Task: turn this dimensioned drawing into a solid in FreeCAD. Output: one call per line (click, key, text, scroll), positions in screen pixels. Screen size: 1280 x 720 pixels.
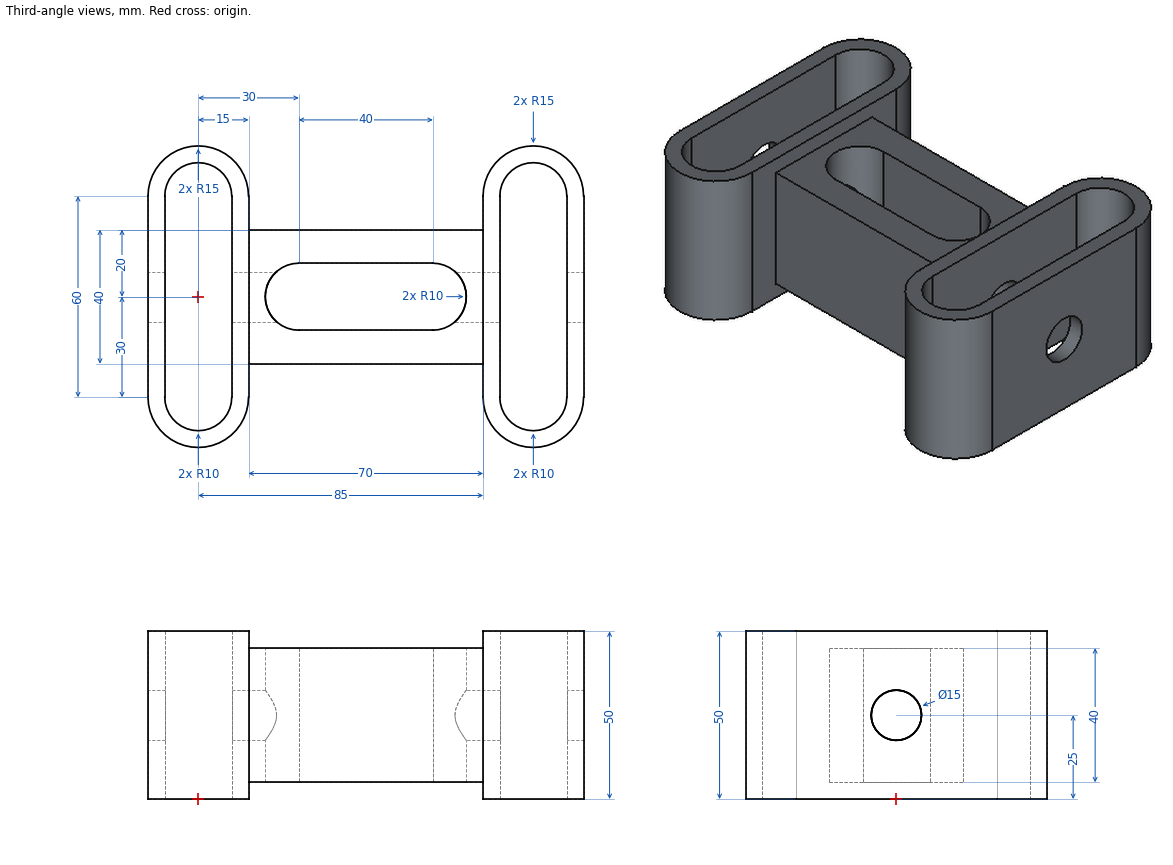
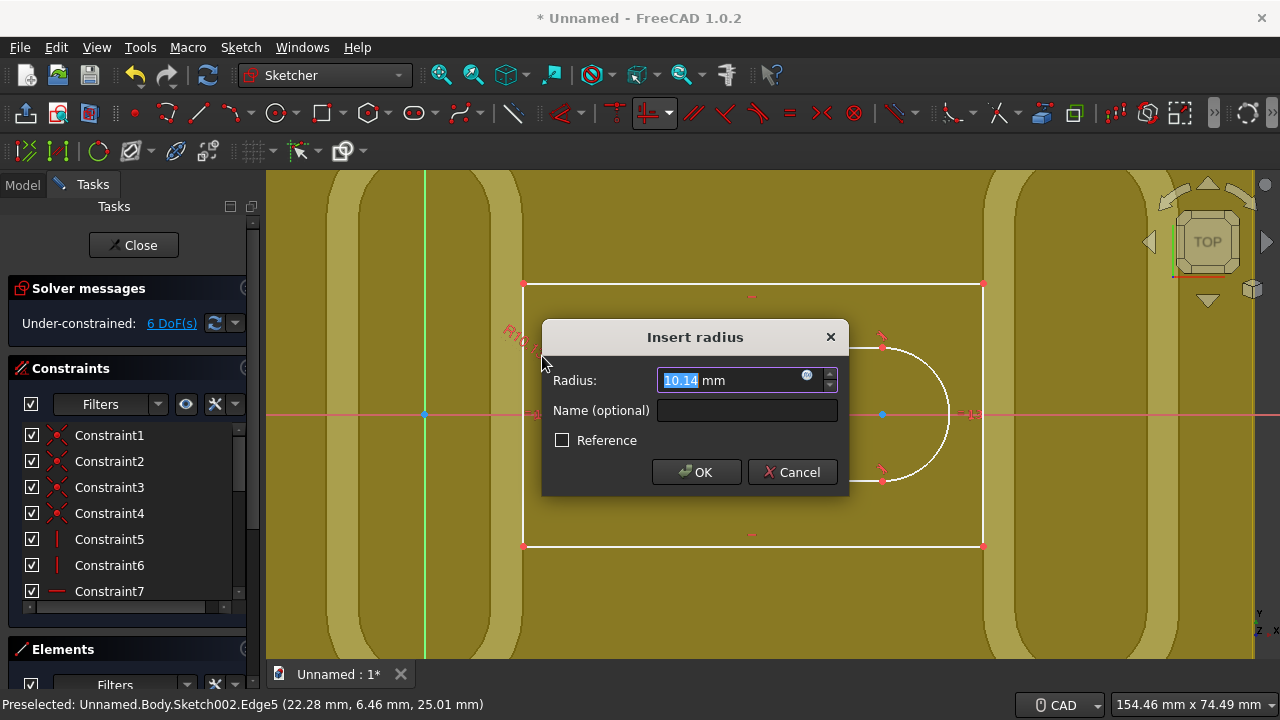
text(10)
key(Return)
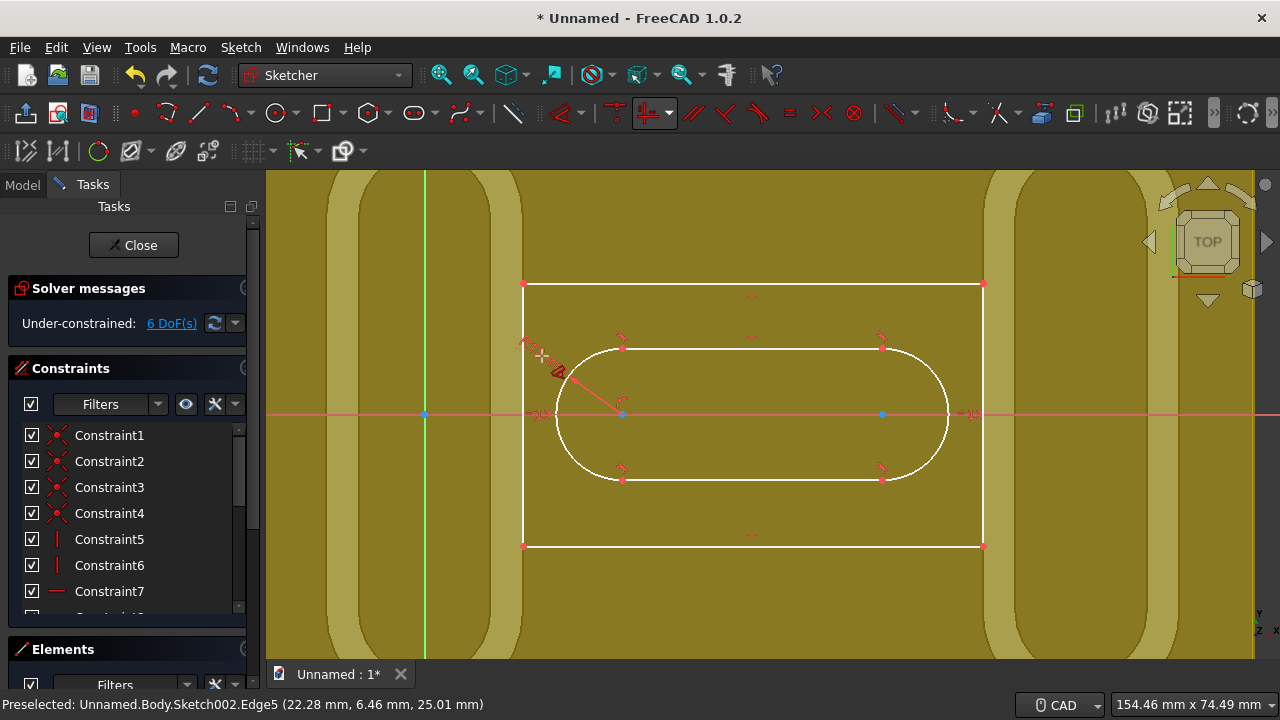
click(523, 363)
click(489, 476)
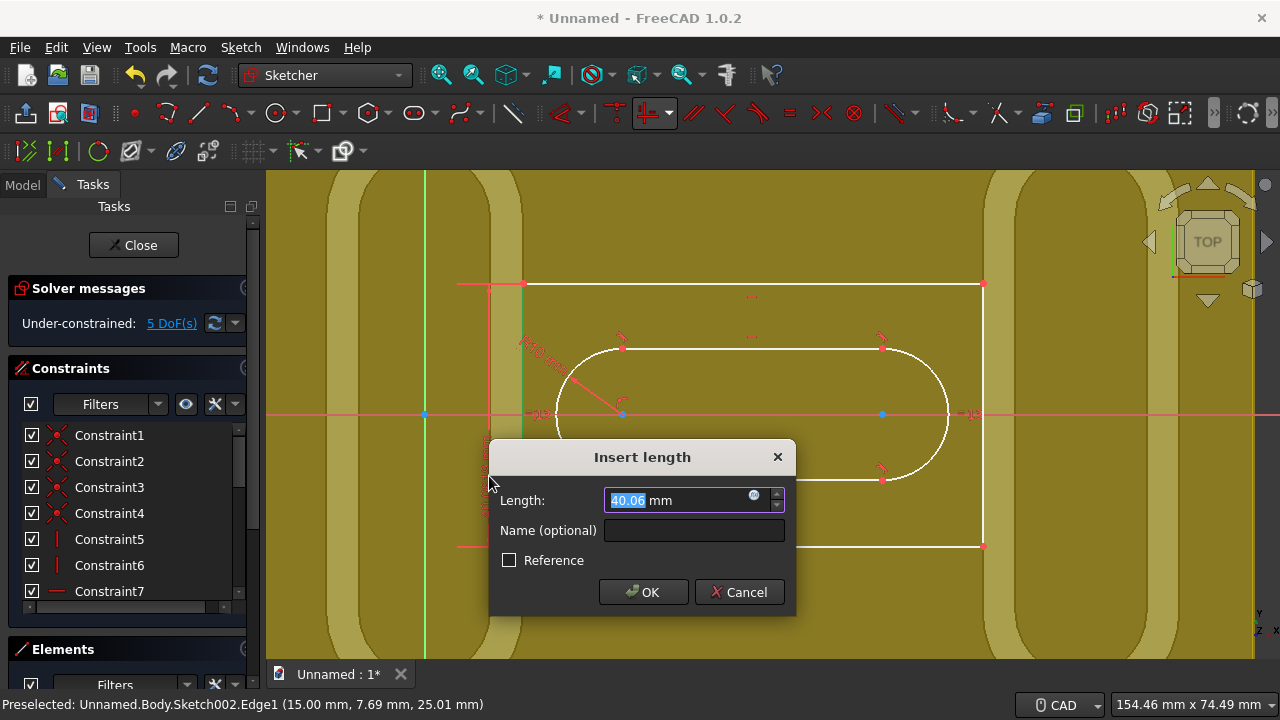
text(40)
key(Return)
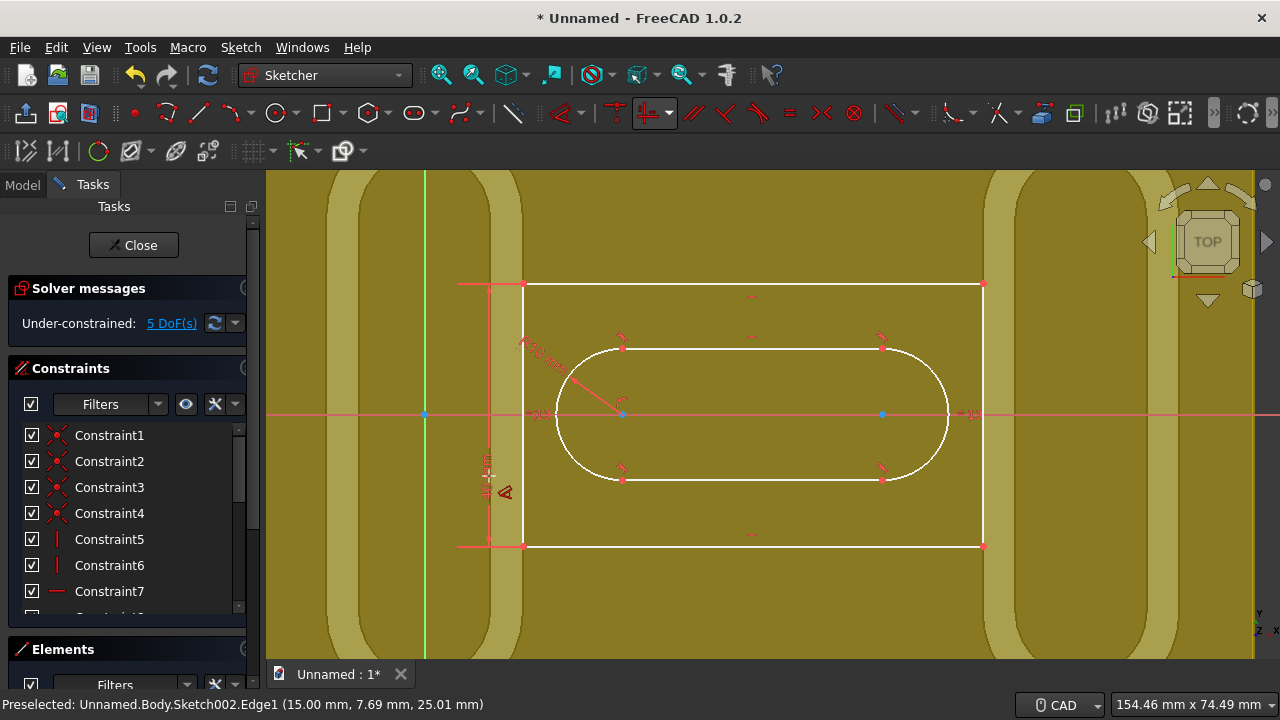
click(661, 547)
click(753, 581)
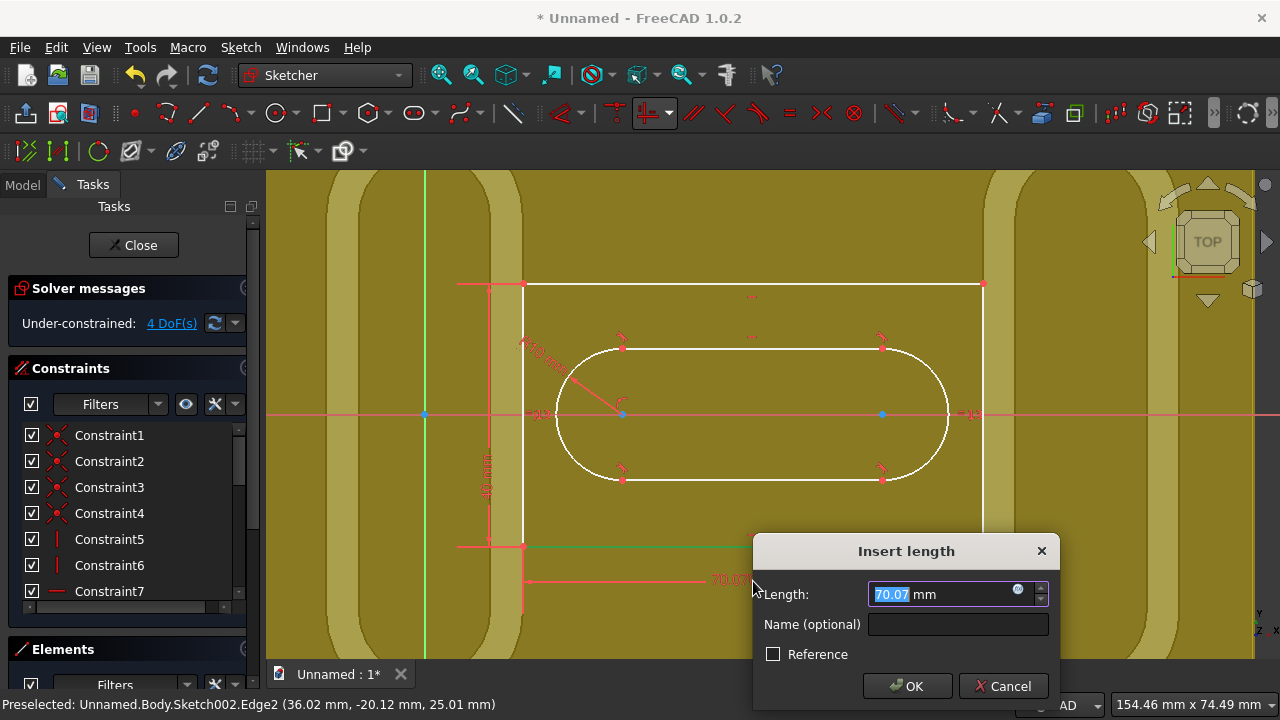
text(70)
key(Return)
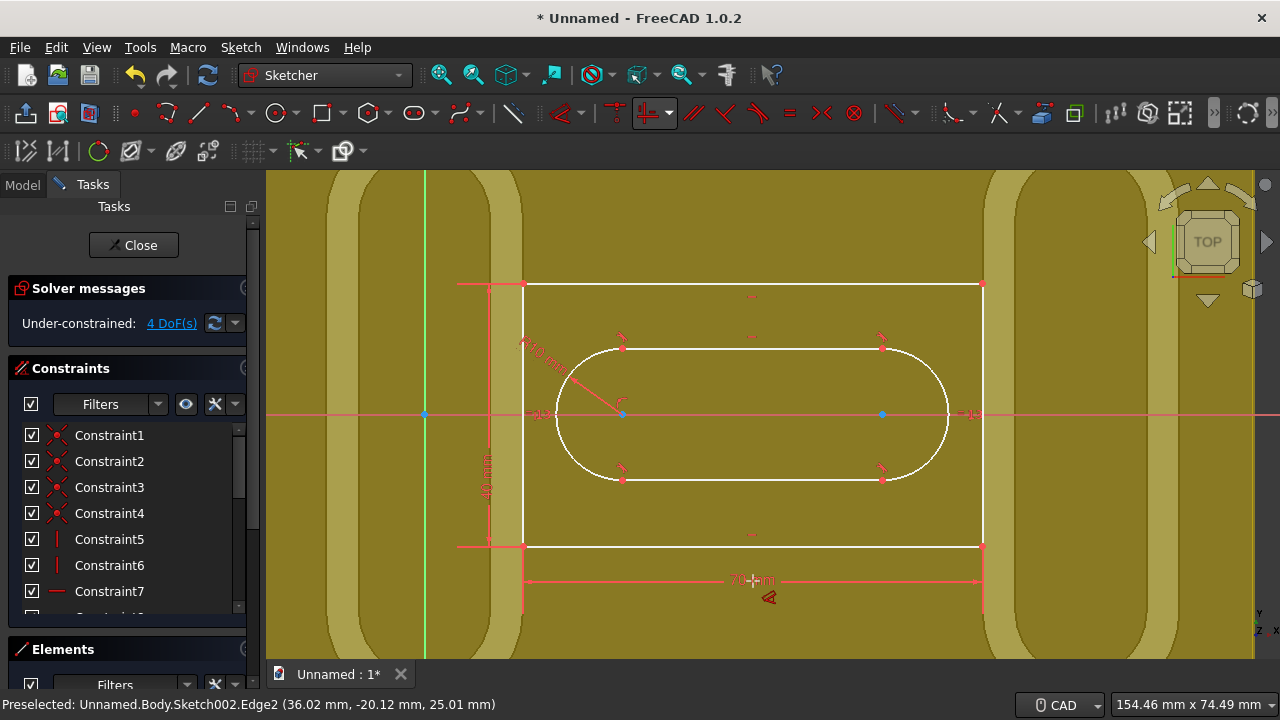
click(700, 349)
click(752, 315)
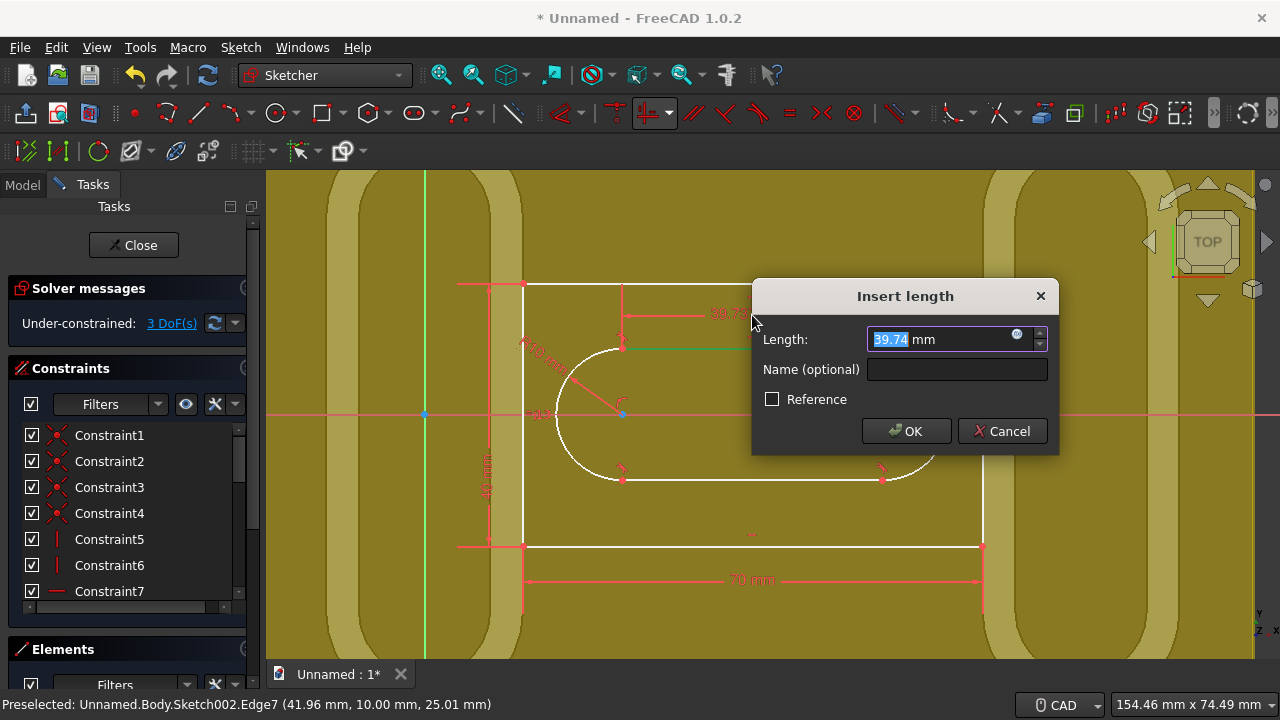
text(40)
key(Return)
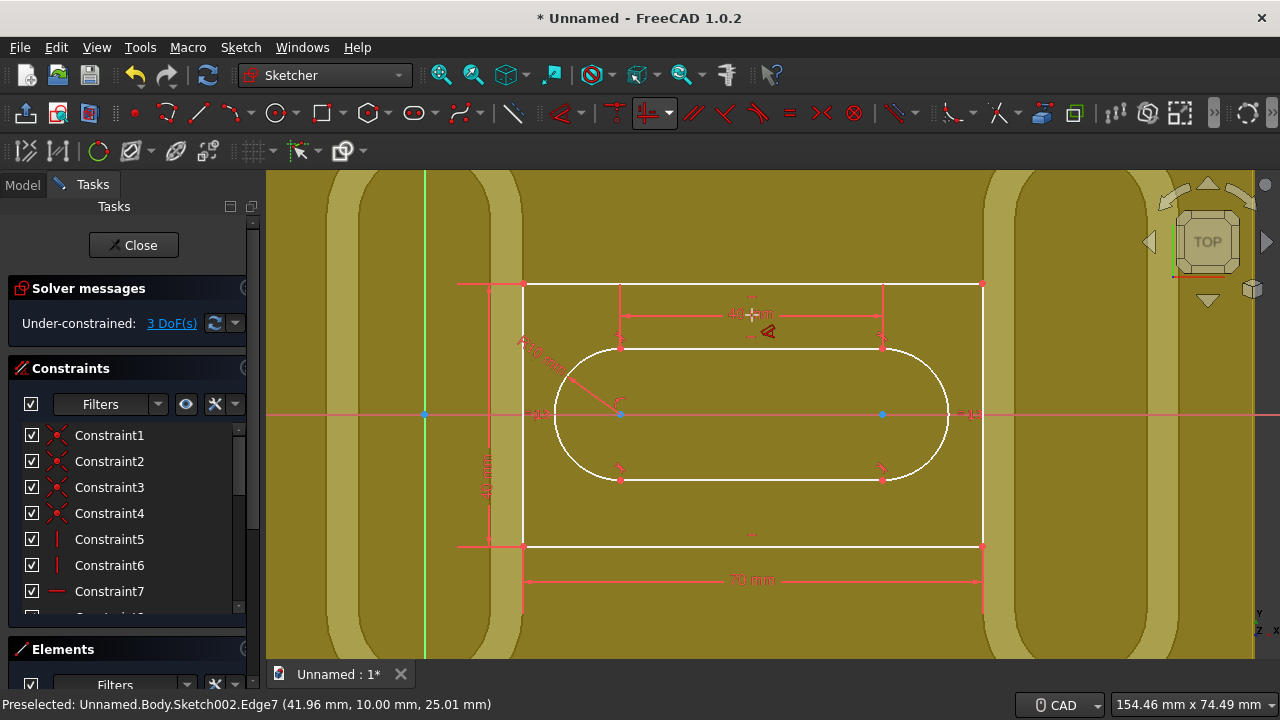
click(523, 284)
click(474, 250)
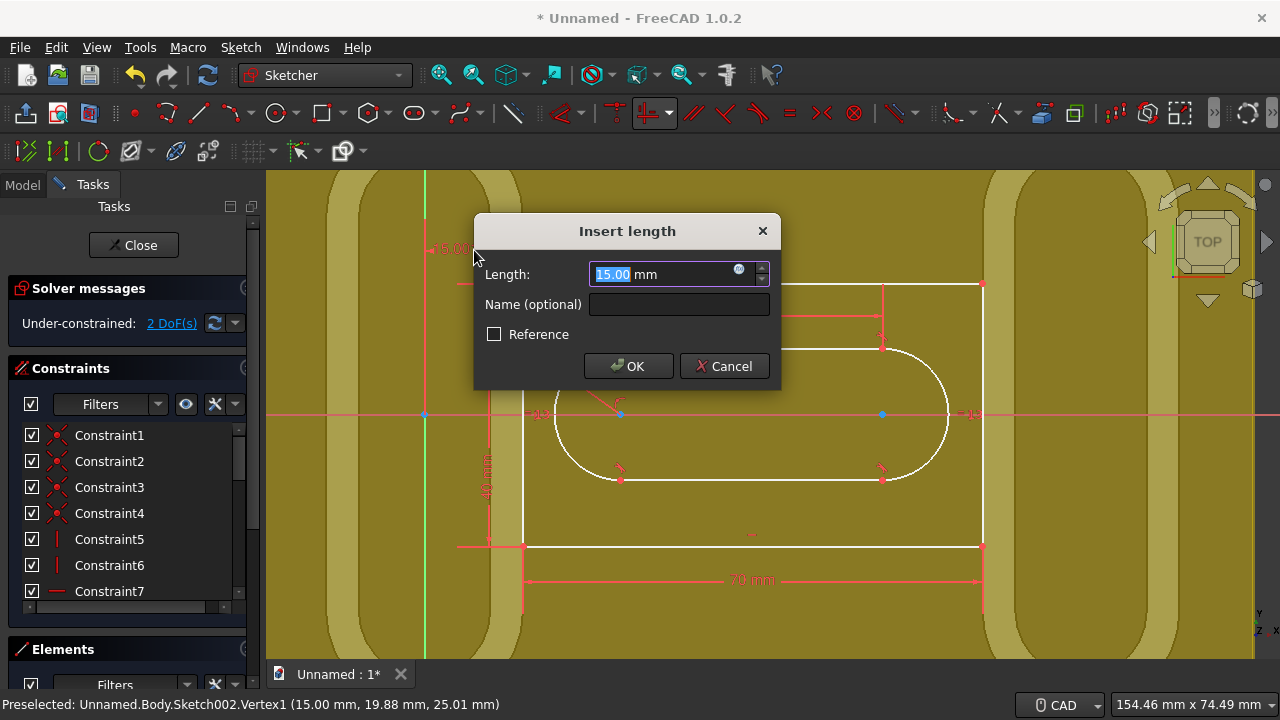
text(15)
key(Return)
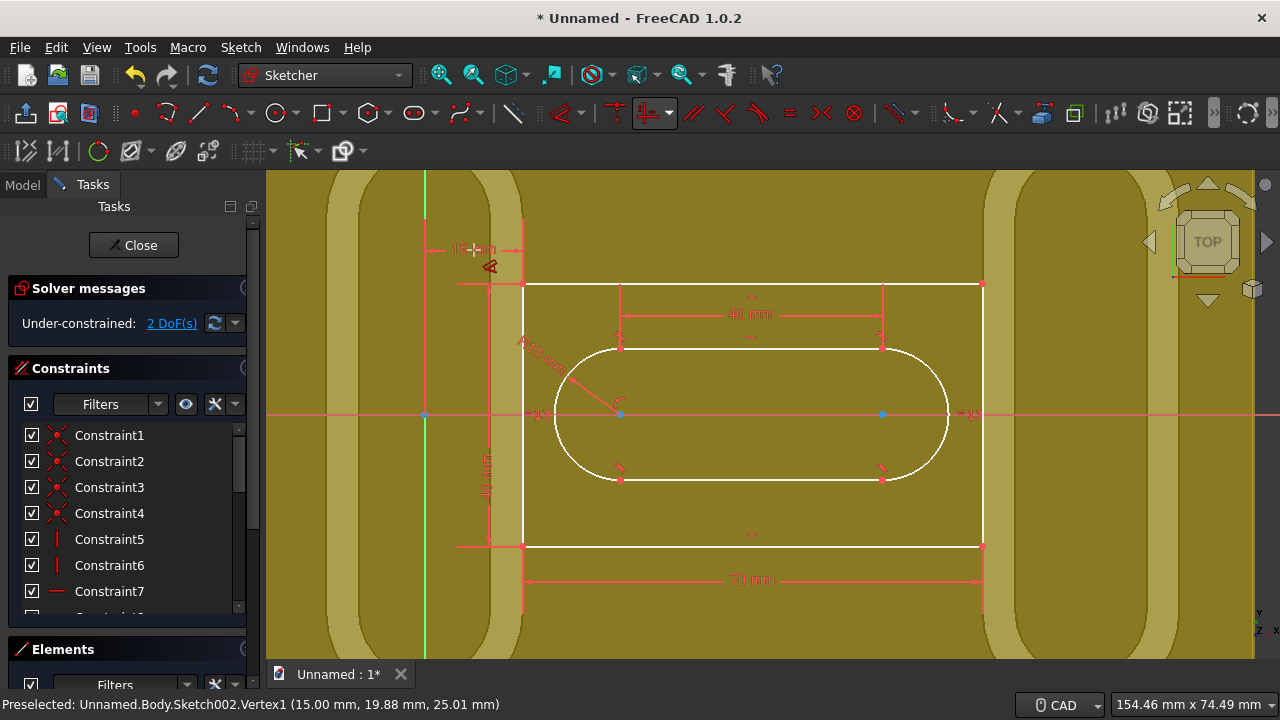
click(523, 284)
click(391, 349)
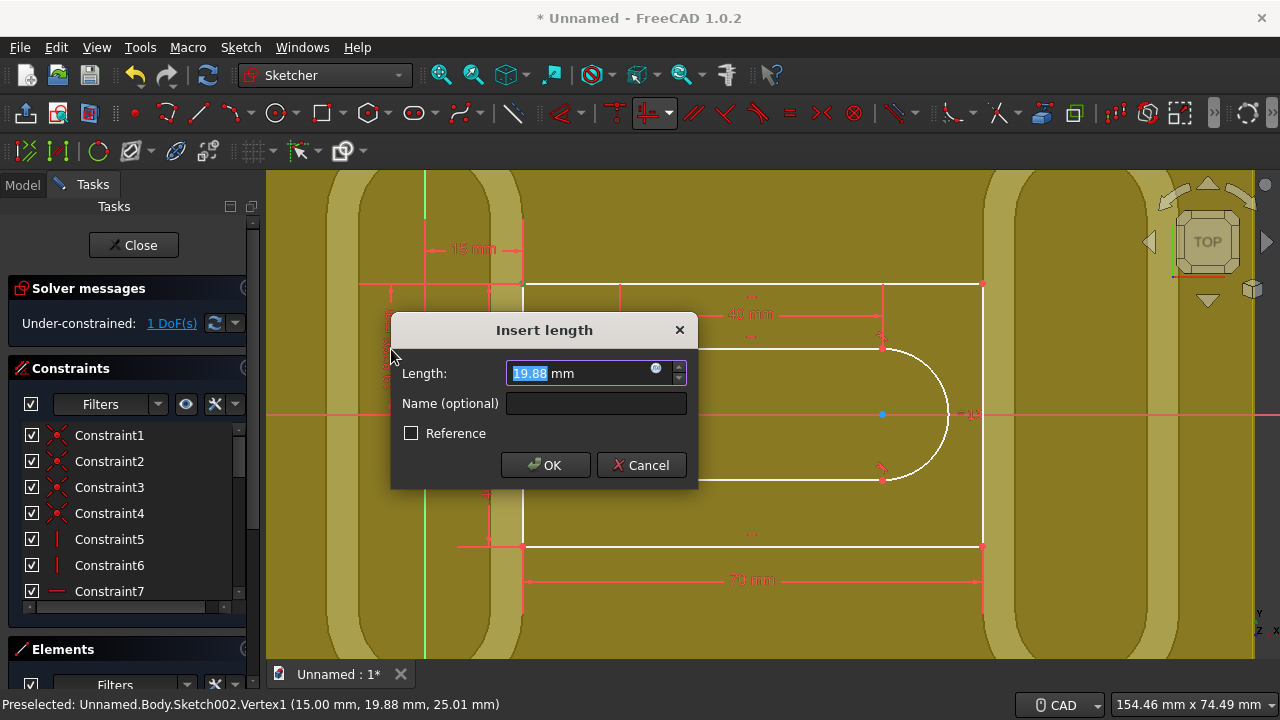
text(20)
key(Return)